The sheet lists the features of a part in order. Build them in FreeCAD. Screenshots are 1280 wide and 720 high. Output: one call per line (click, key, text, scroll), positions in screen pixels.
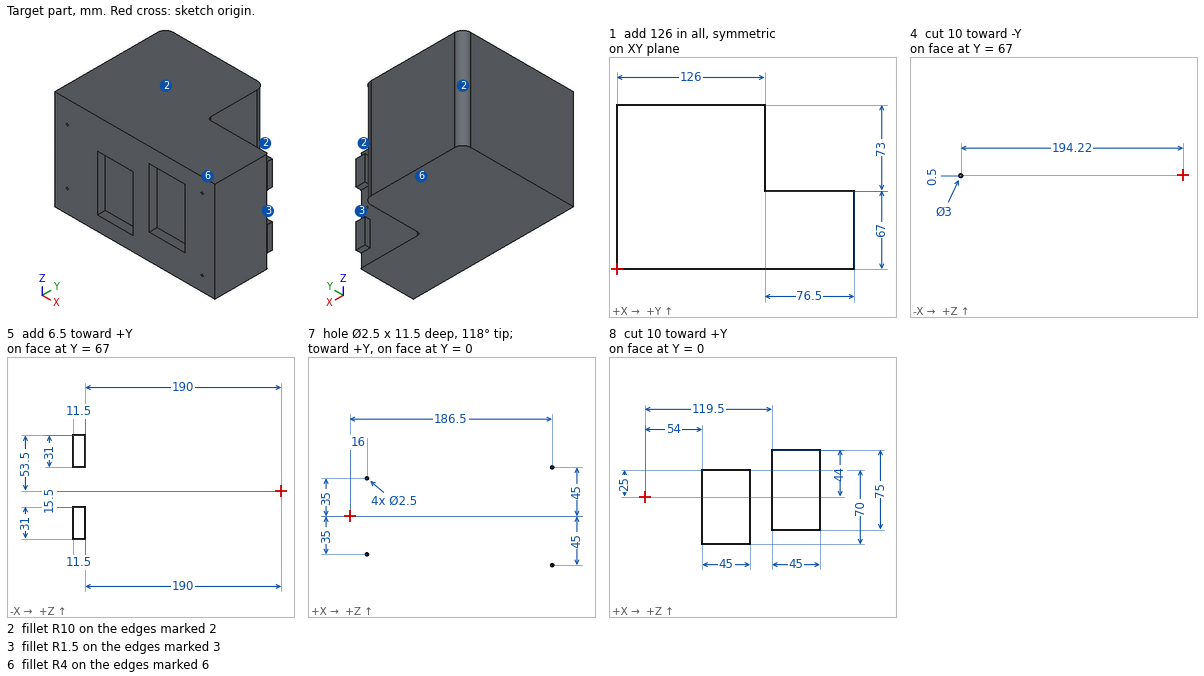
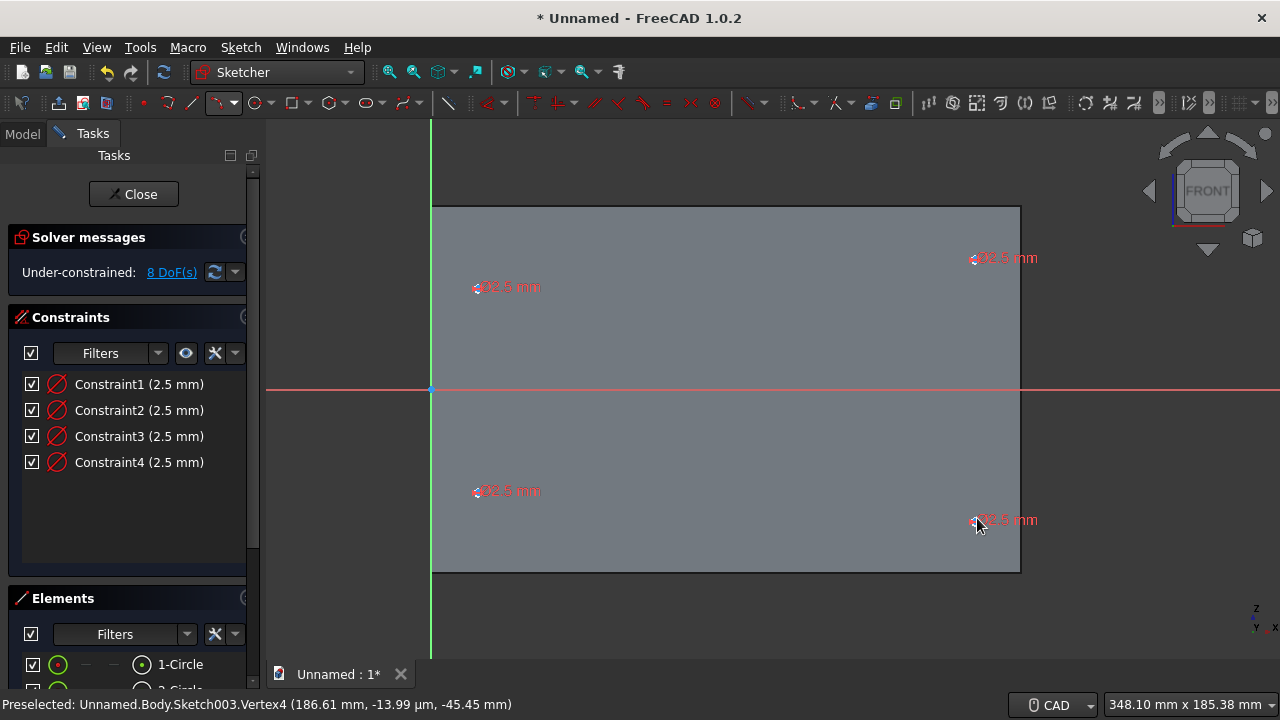
click(478, 289)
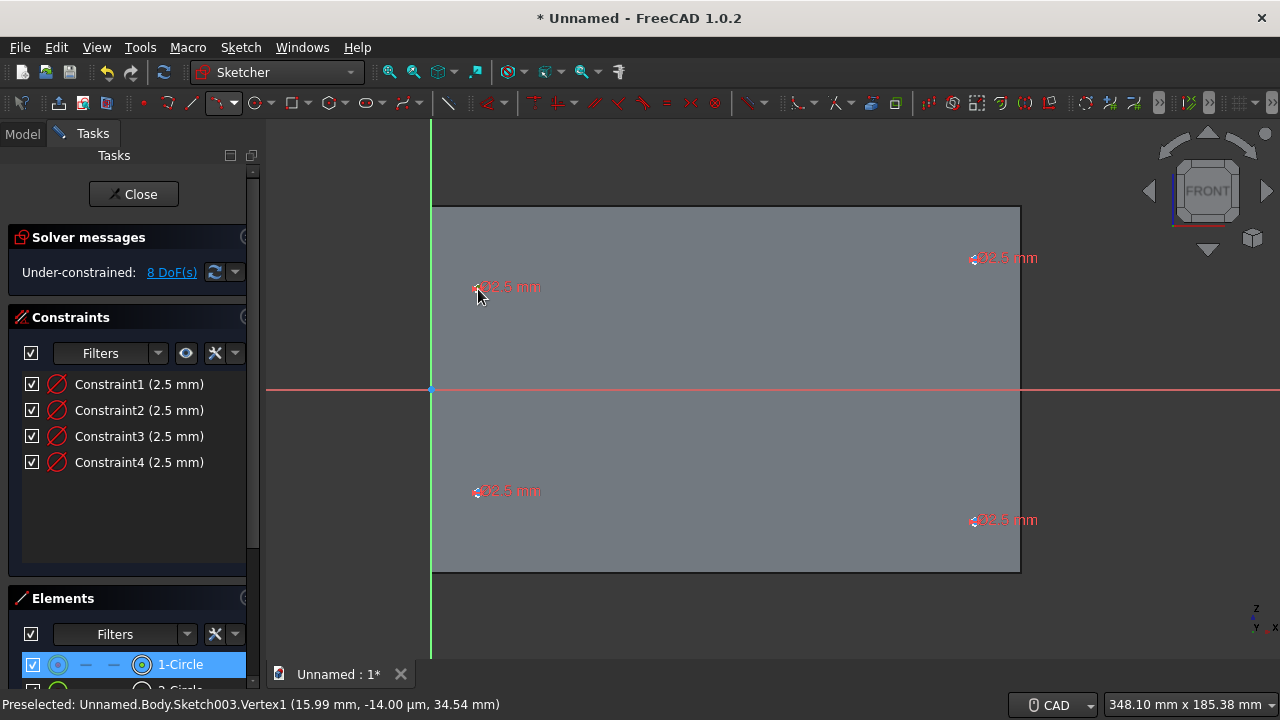
click(478, 493)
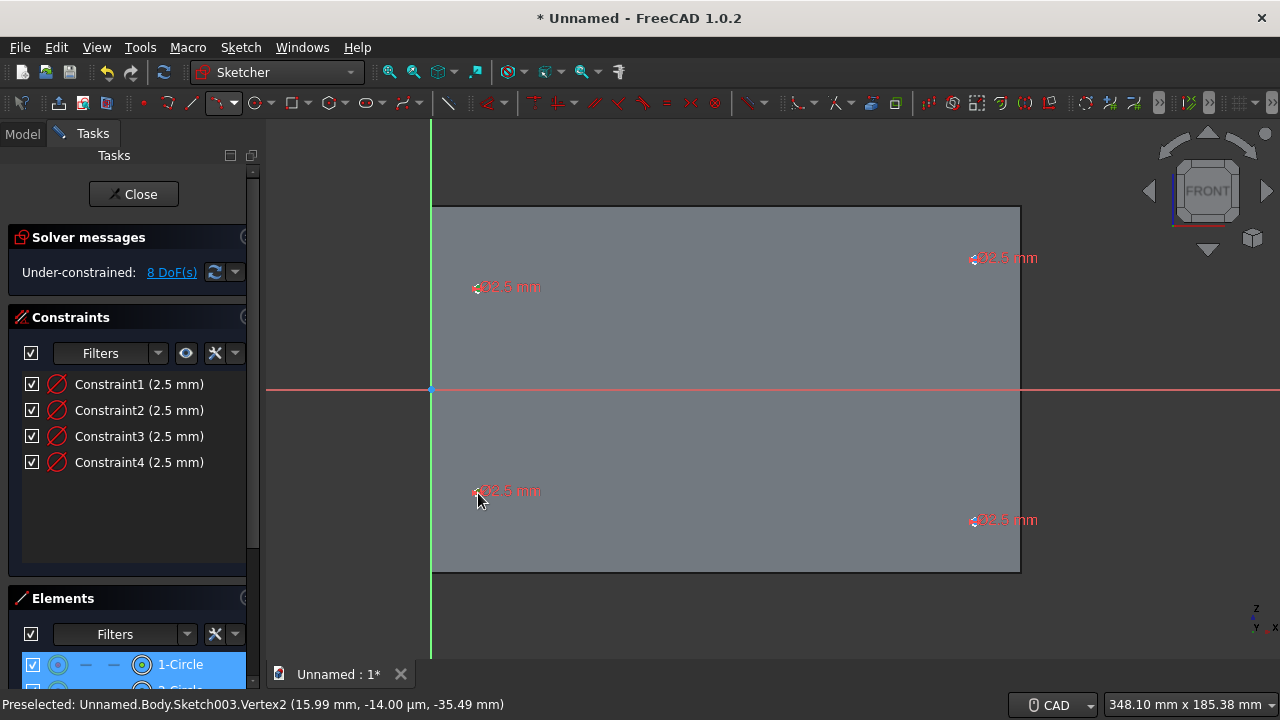
key(v)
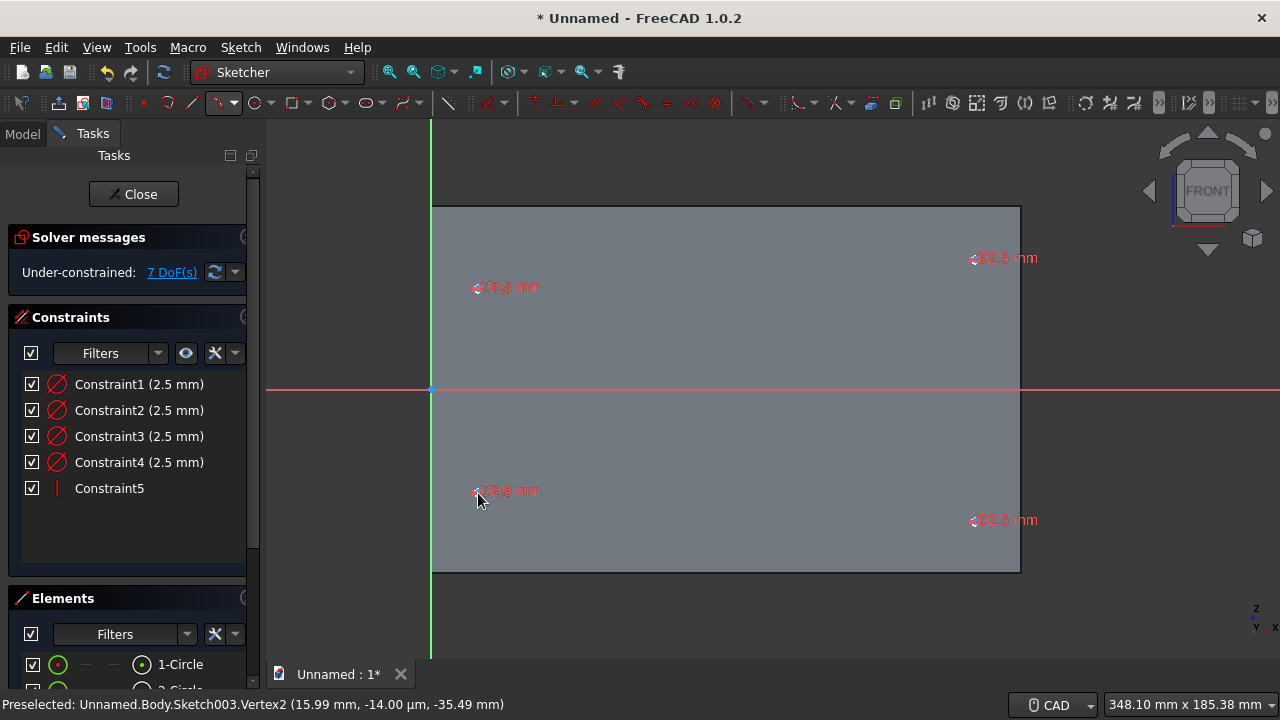
click(975, 260)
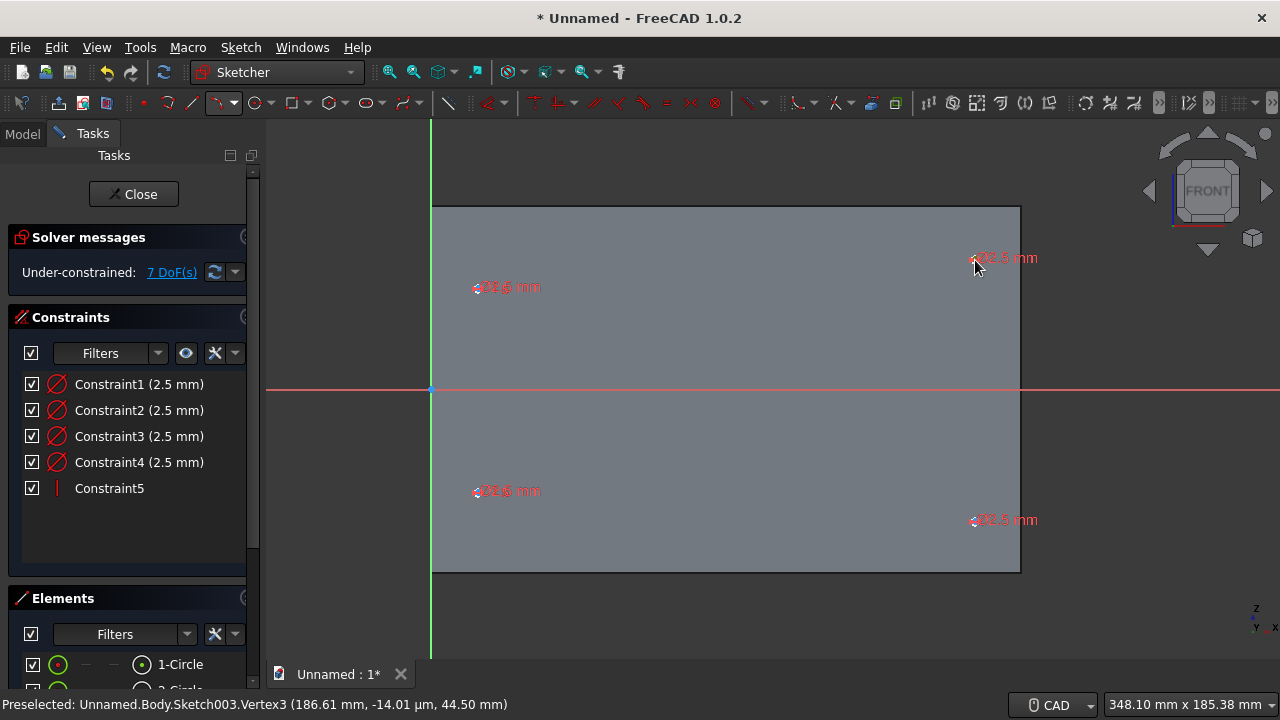
click(975, 522)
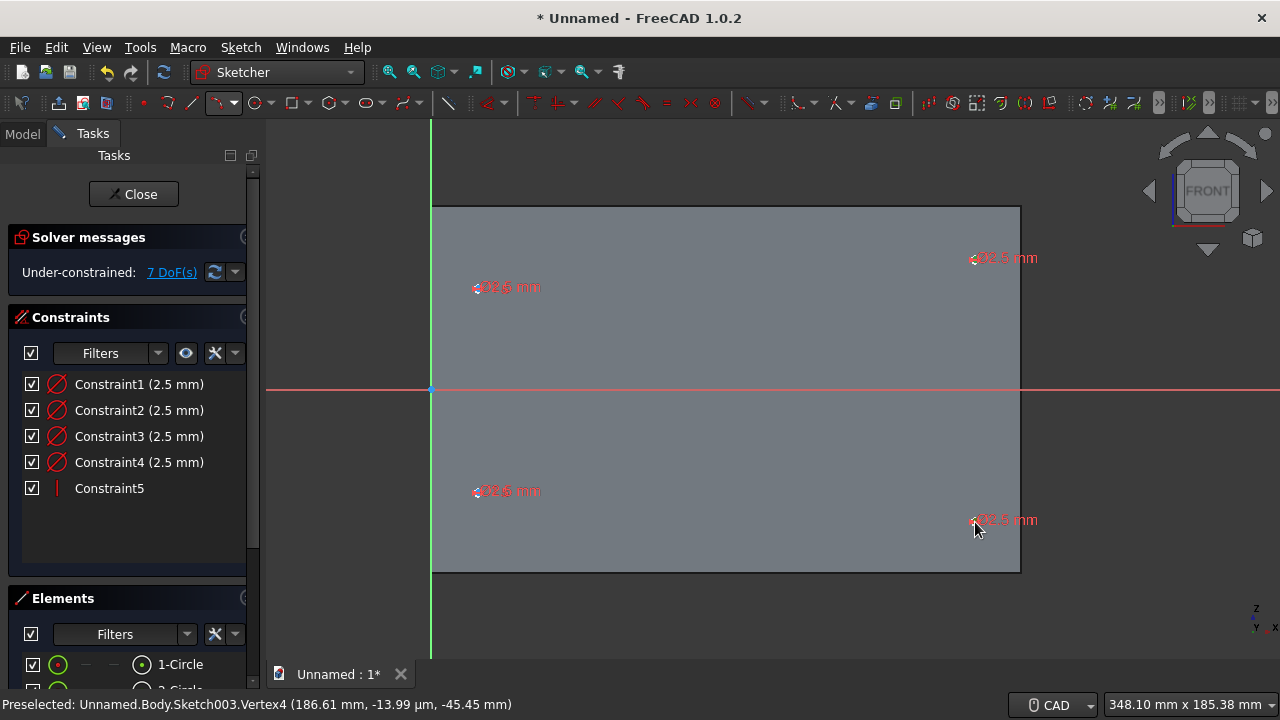
key(v)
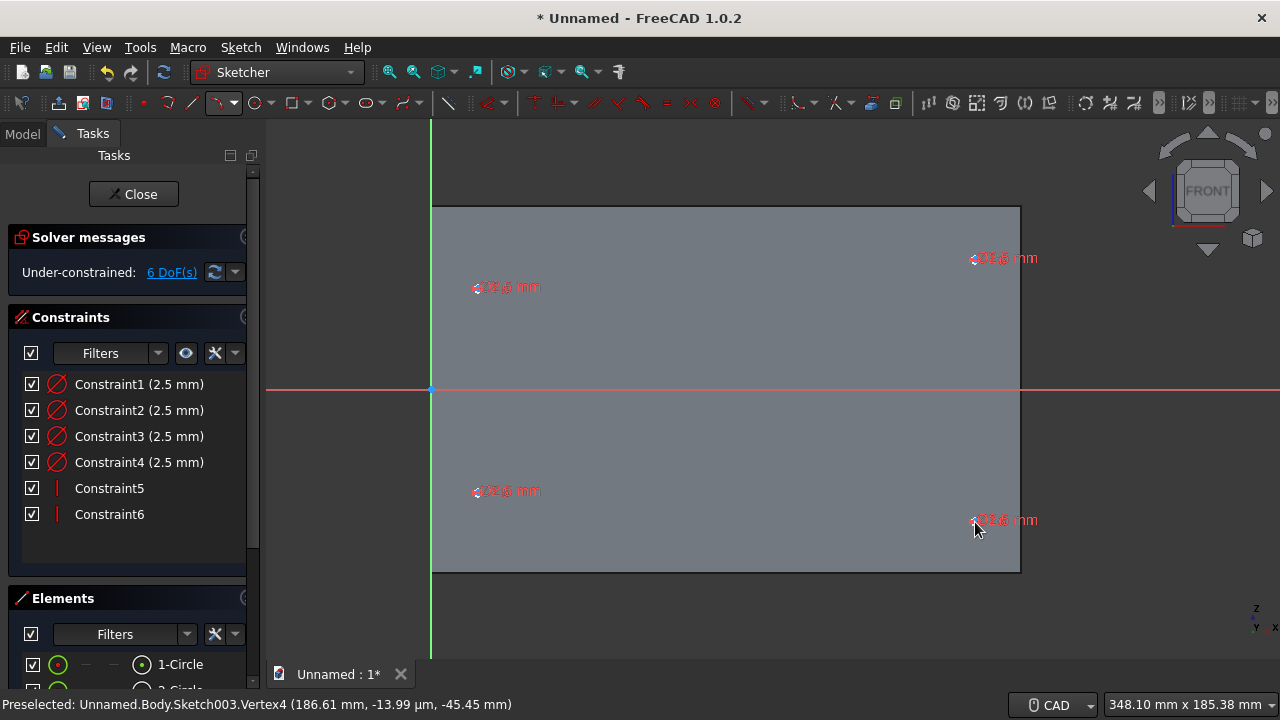
key(d)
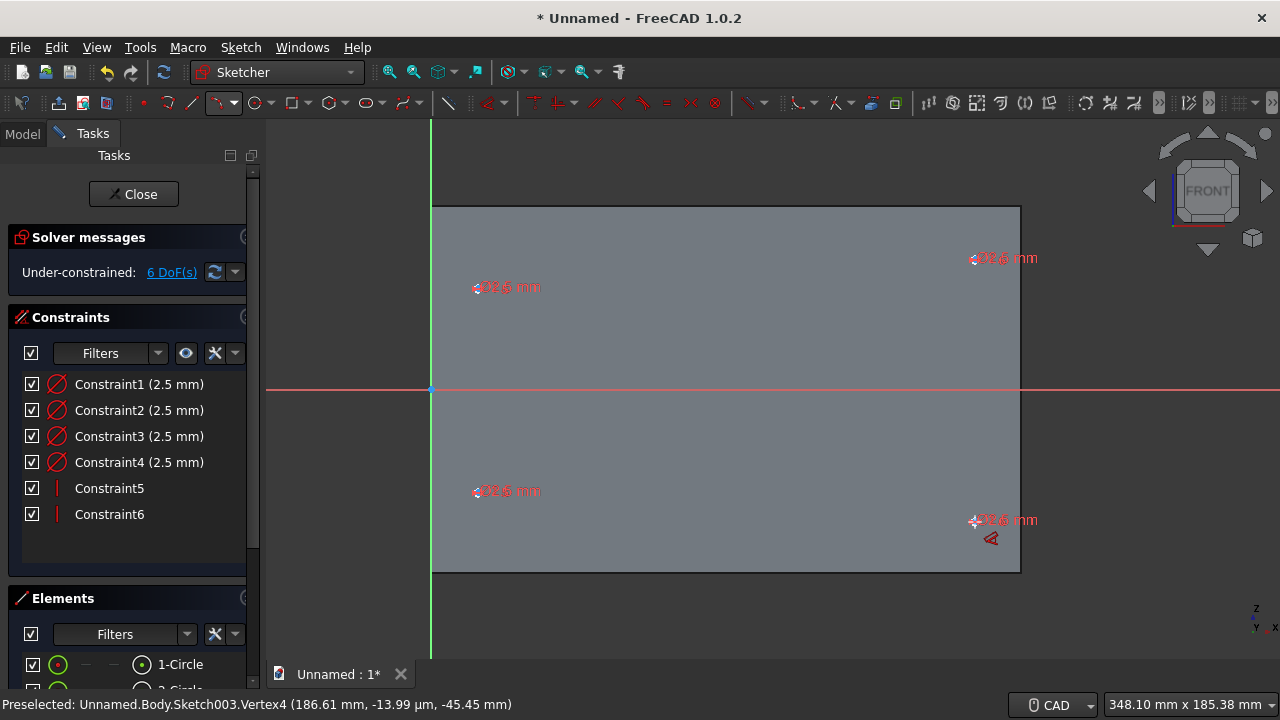
click(478, 289)
click(455, 255)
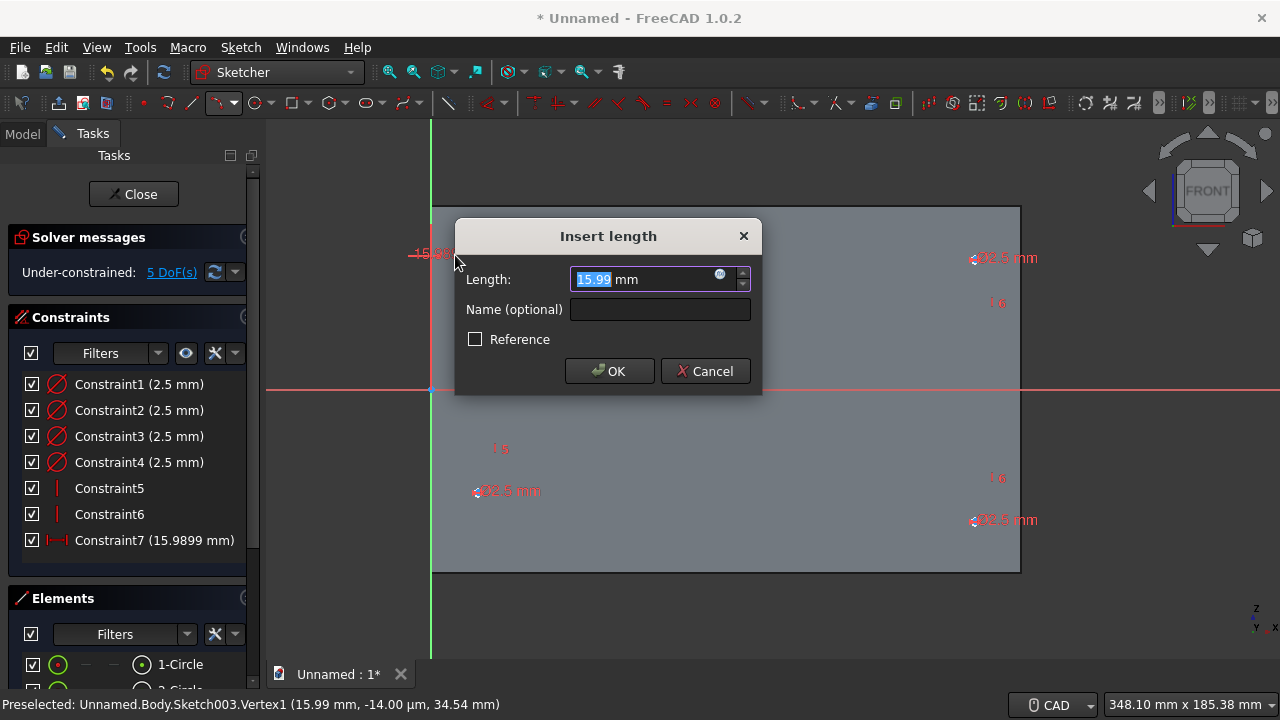
text(16)
key(Return)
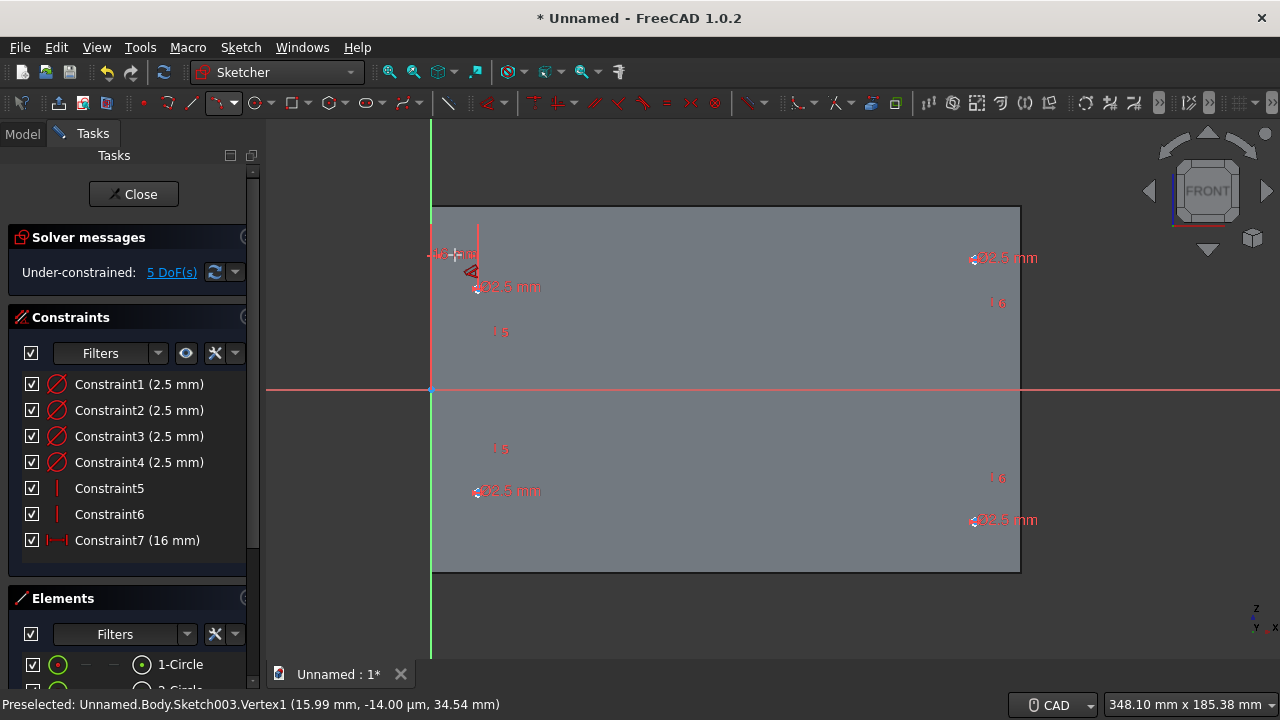
click(478, 289)
click(397, 339)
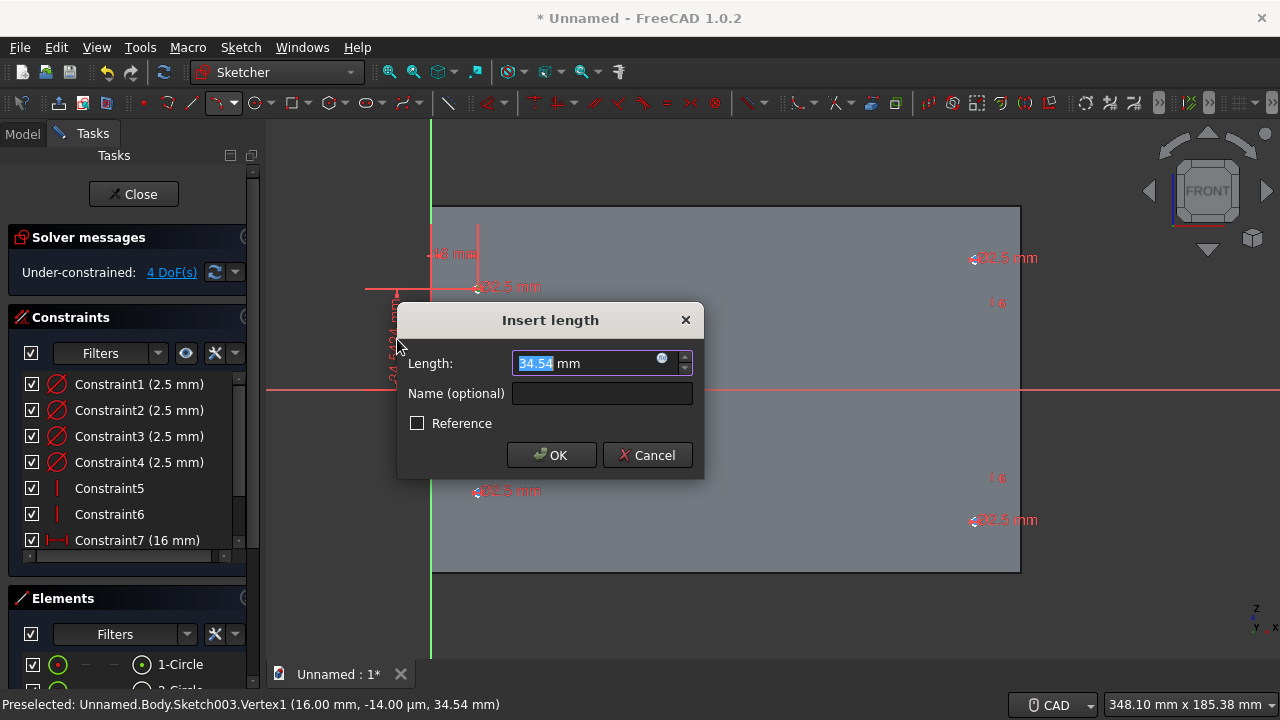
text(35)
key(Return)